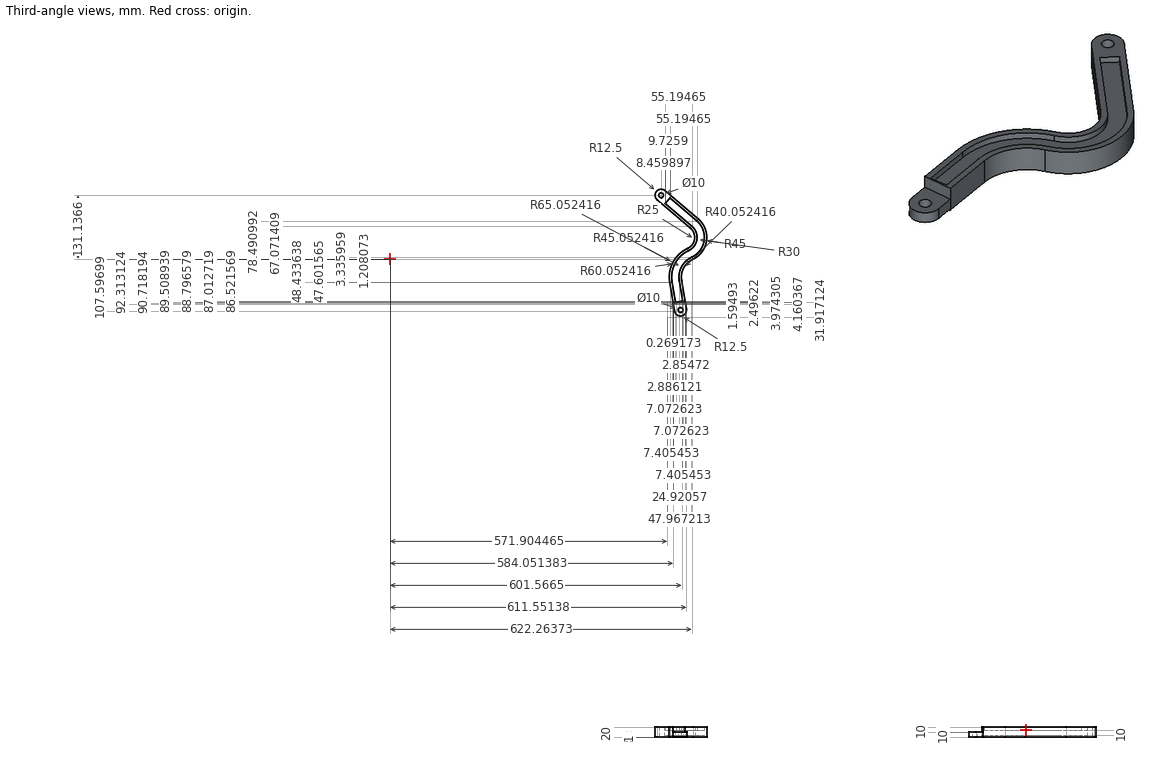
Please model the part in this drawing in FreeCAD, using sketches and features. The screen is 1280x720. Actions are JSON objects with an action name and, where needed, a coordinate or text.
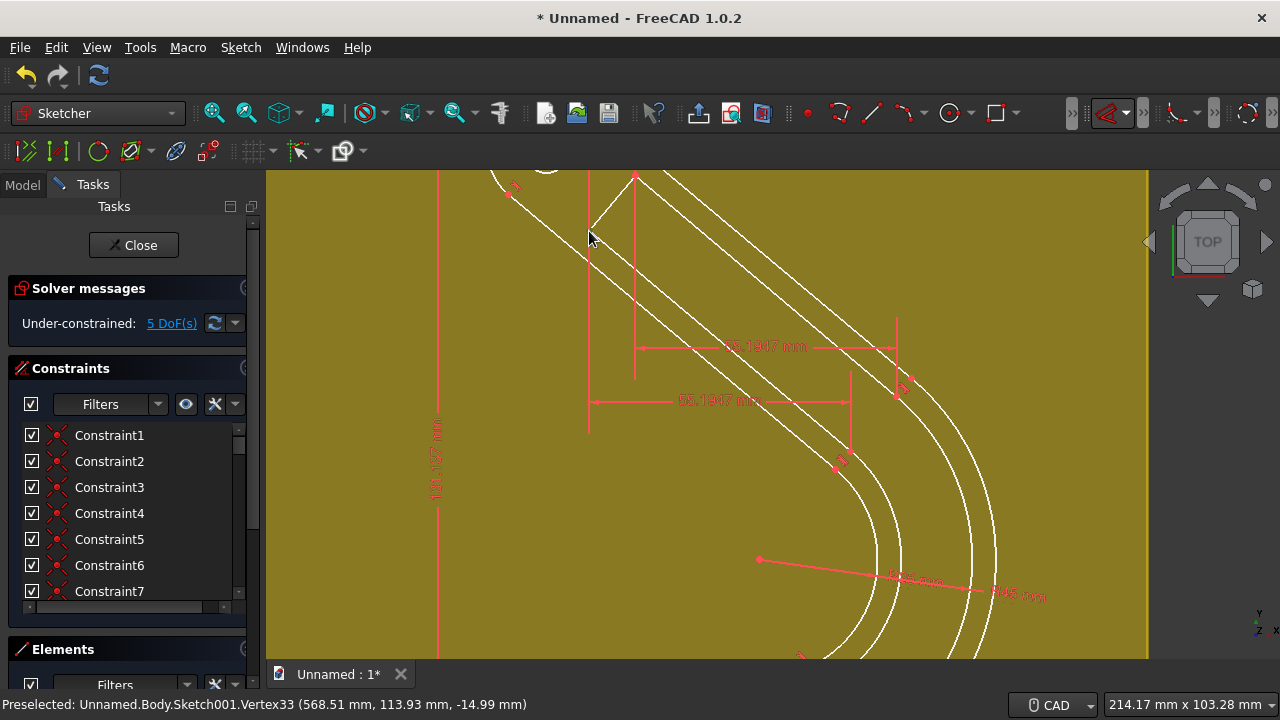
{"action": "scroll", "coordinate": [687, 311], "scroll_direction": "down", "scroll_amount": 6}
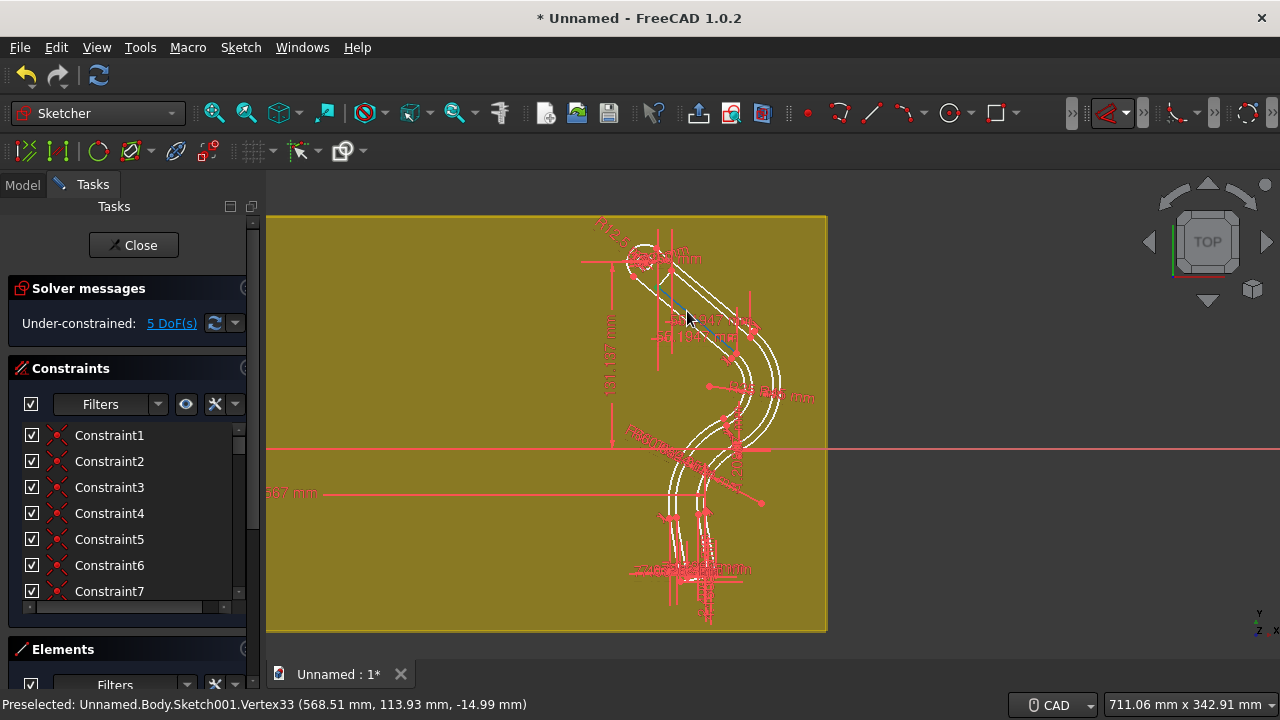
{"action": "scroll", "coordinate": [645, 262], "scroll_direction": "up", "scroll_amount": 6}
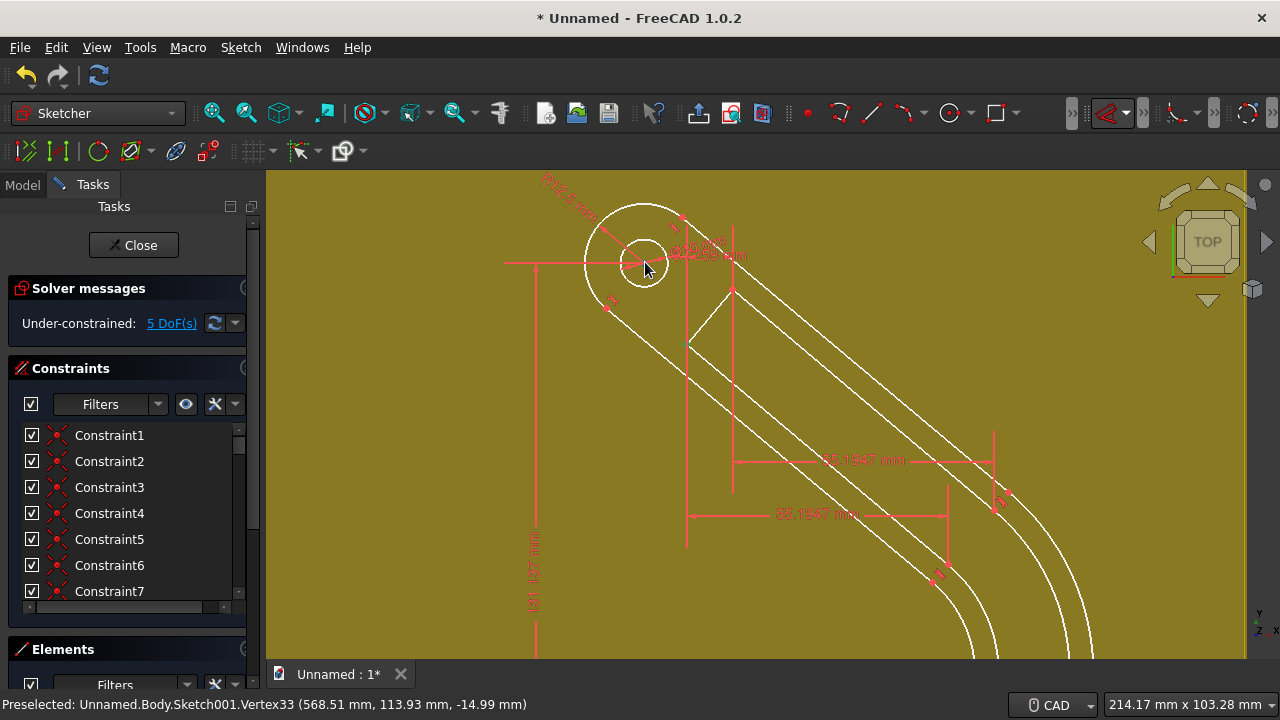
{"action": "left_click", "coordinate": [644, 263]}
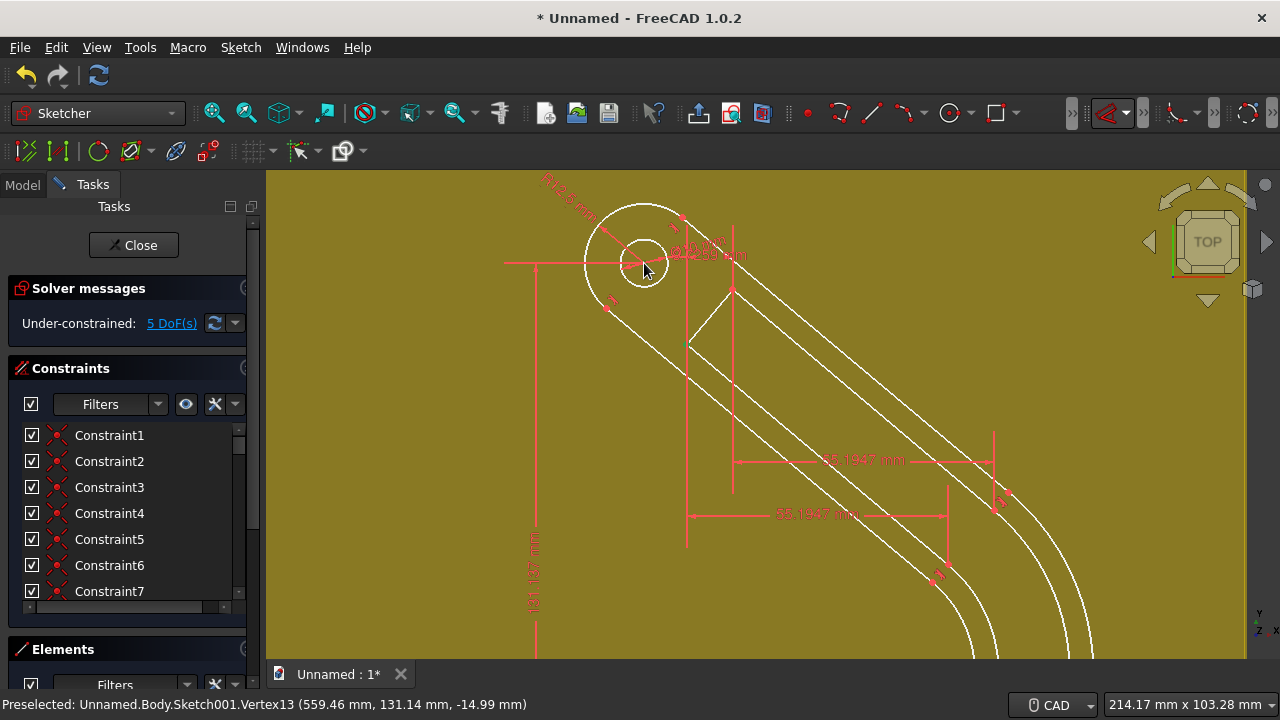
{"action": "left_click", "coordinate": [1128, 114]}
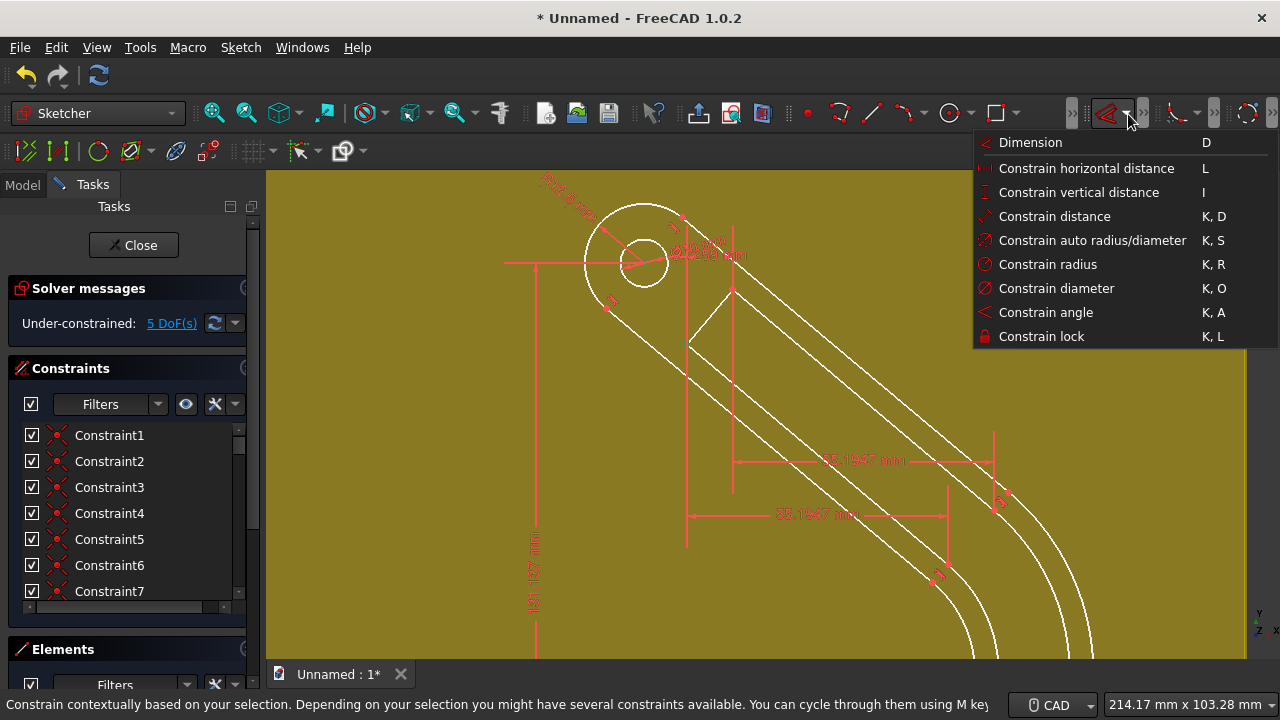
{"action": "left_click", "coordinate": [1126, 168]}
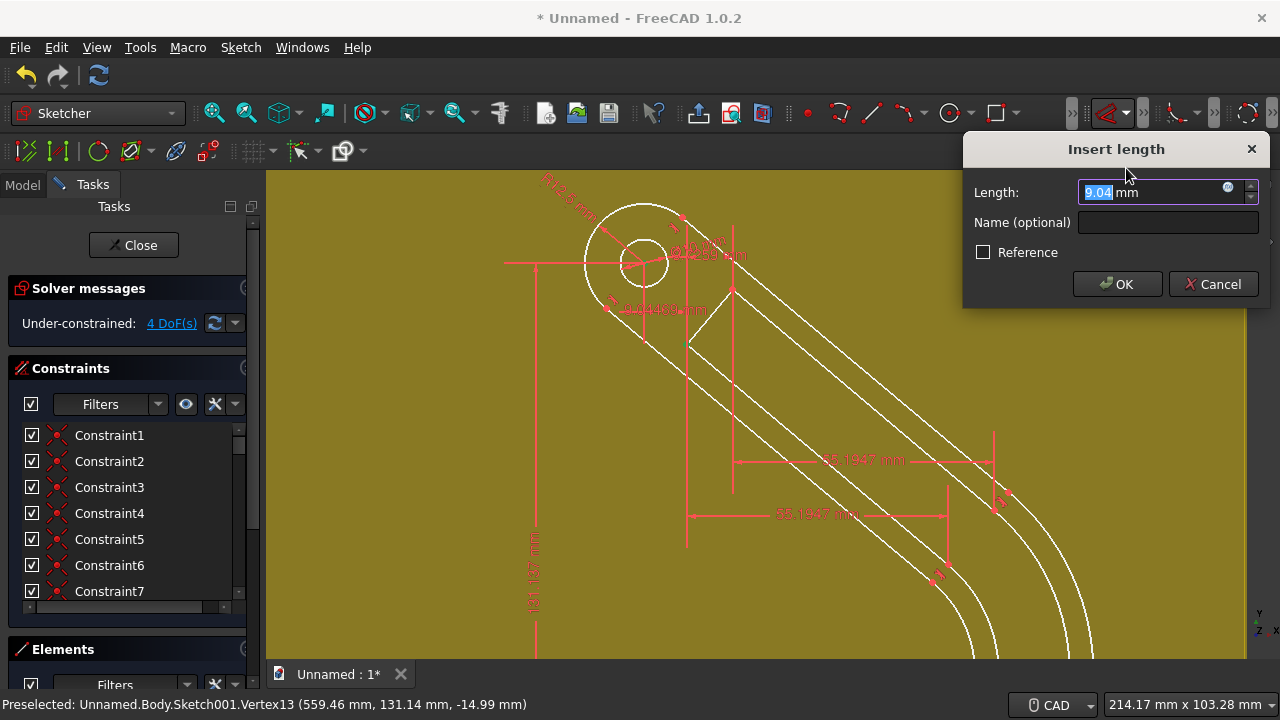
{"action": "type", "text": "8.459897"}
{"action": "key", "text": "Return"}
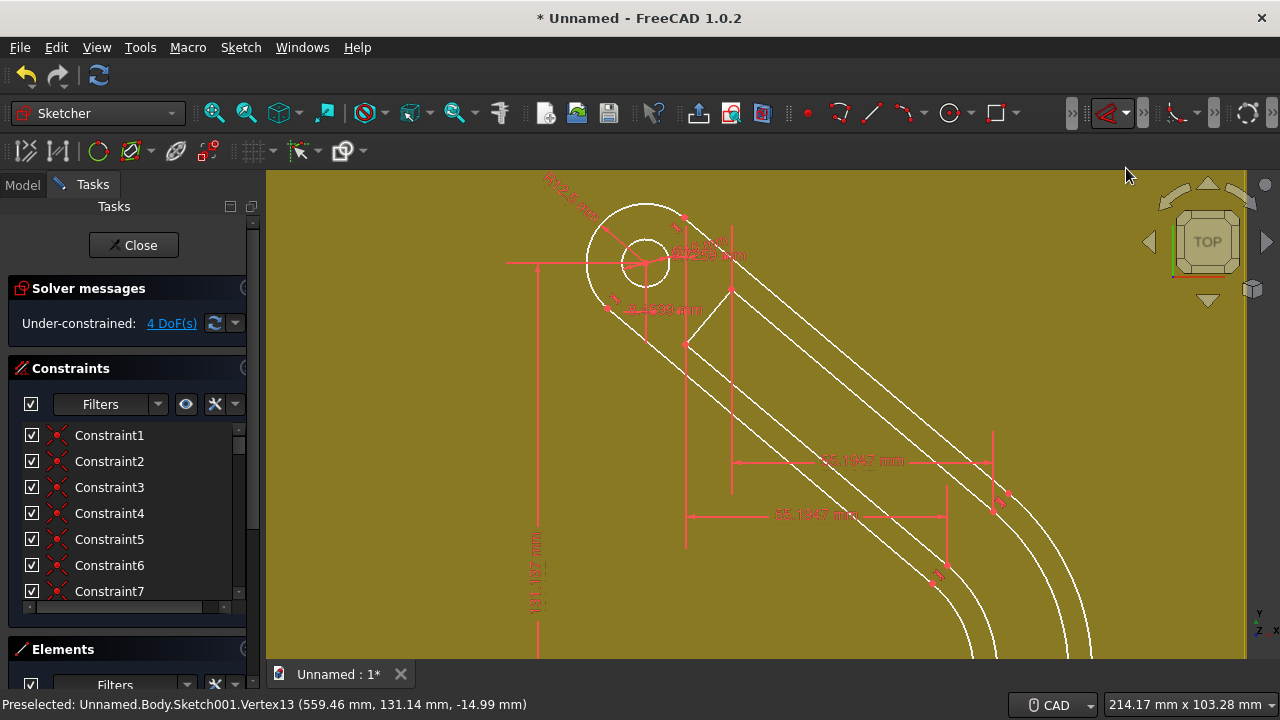
{"action": "scroll", "coordinate": [645, 261], "scroll_direction": "down", "scroll_amount": 6}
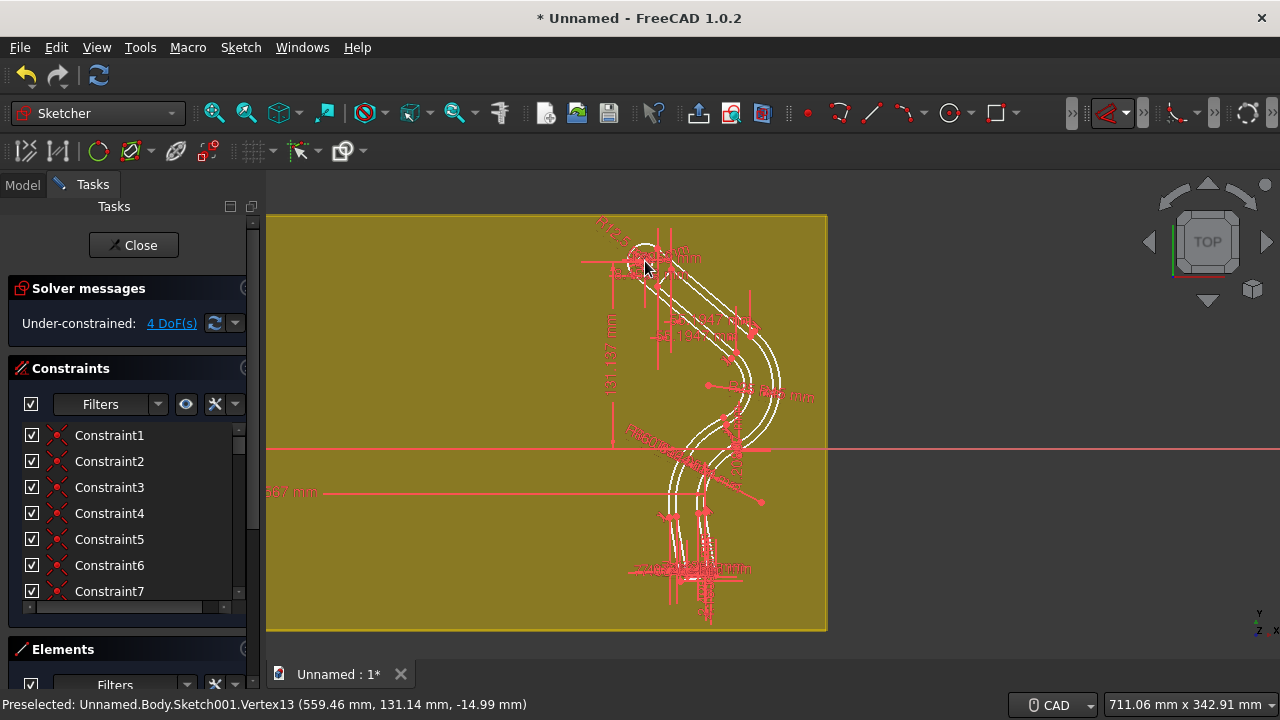
{"action": "scroll", "coordinate": [670, 518], "scroll_direction": "up", "scroll_amount": 3}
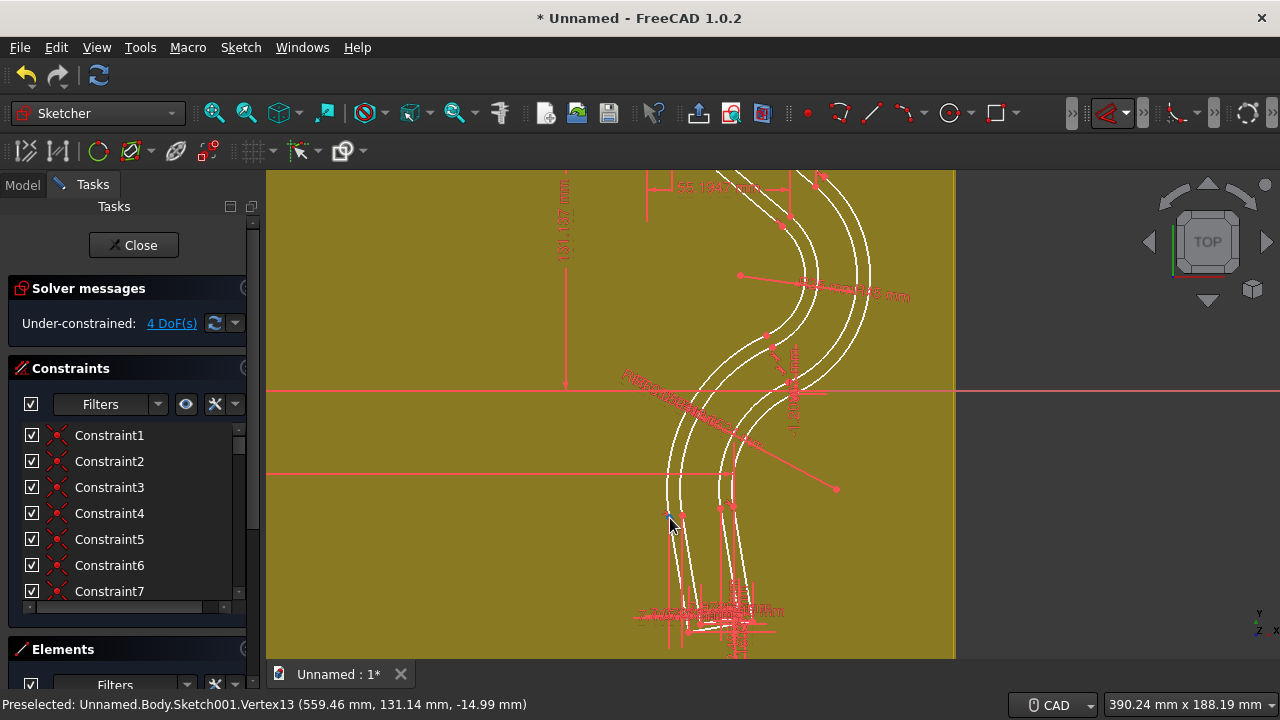
{"action": "left_click", "coordinate": [669, 517]}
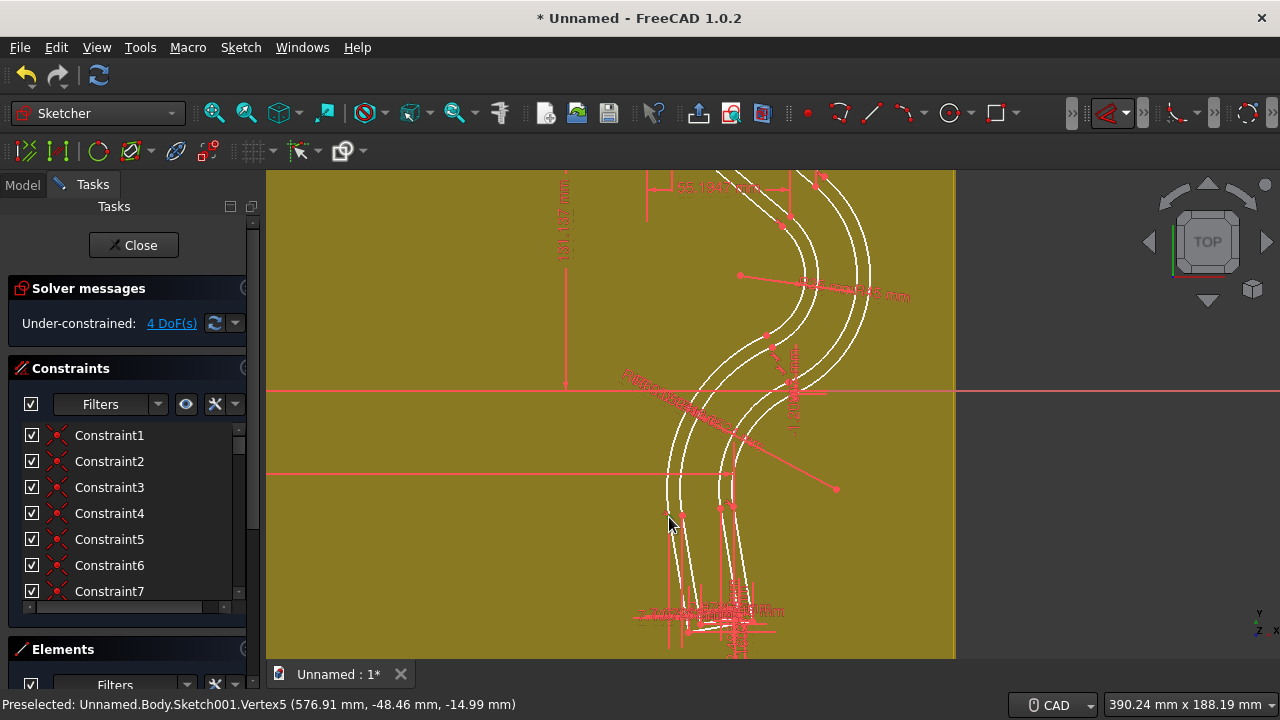
{"action": "left_click", "coordinate": [1128, 114]}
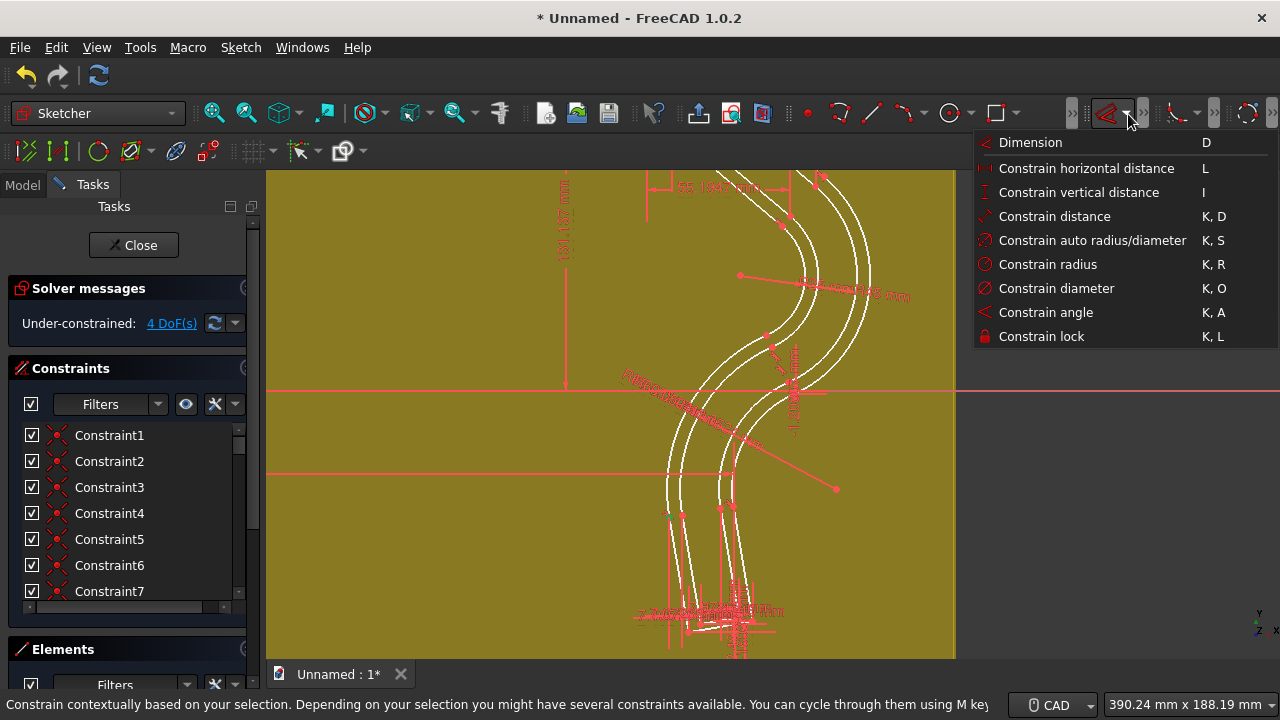
{"action": "left_click", "coordinate": [1126, 192]}